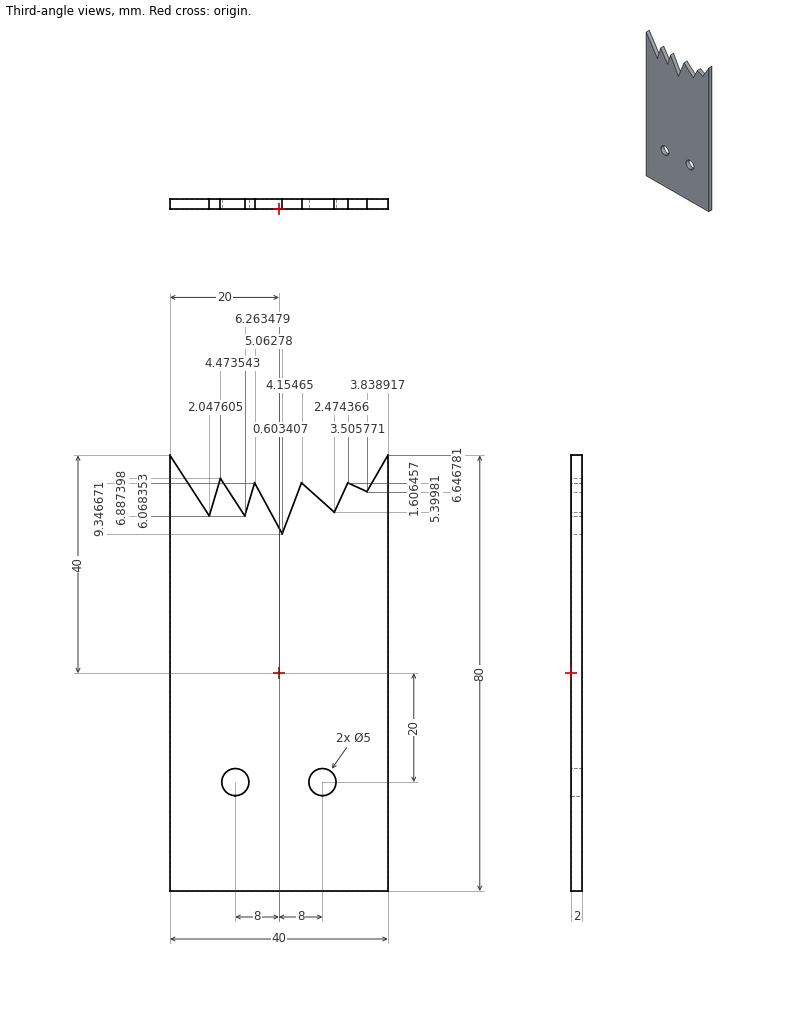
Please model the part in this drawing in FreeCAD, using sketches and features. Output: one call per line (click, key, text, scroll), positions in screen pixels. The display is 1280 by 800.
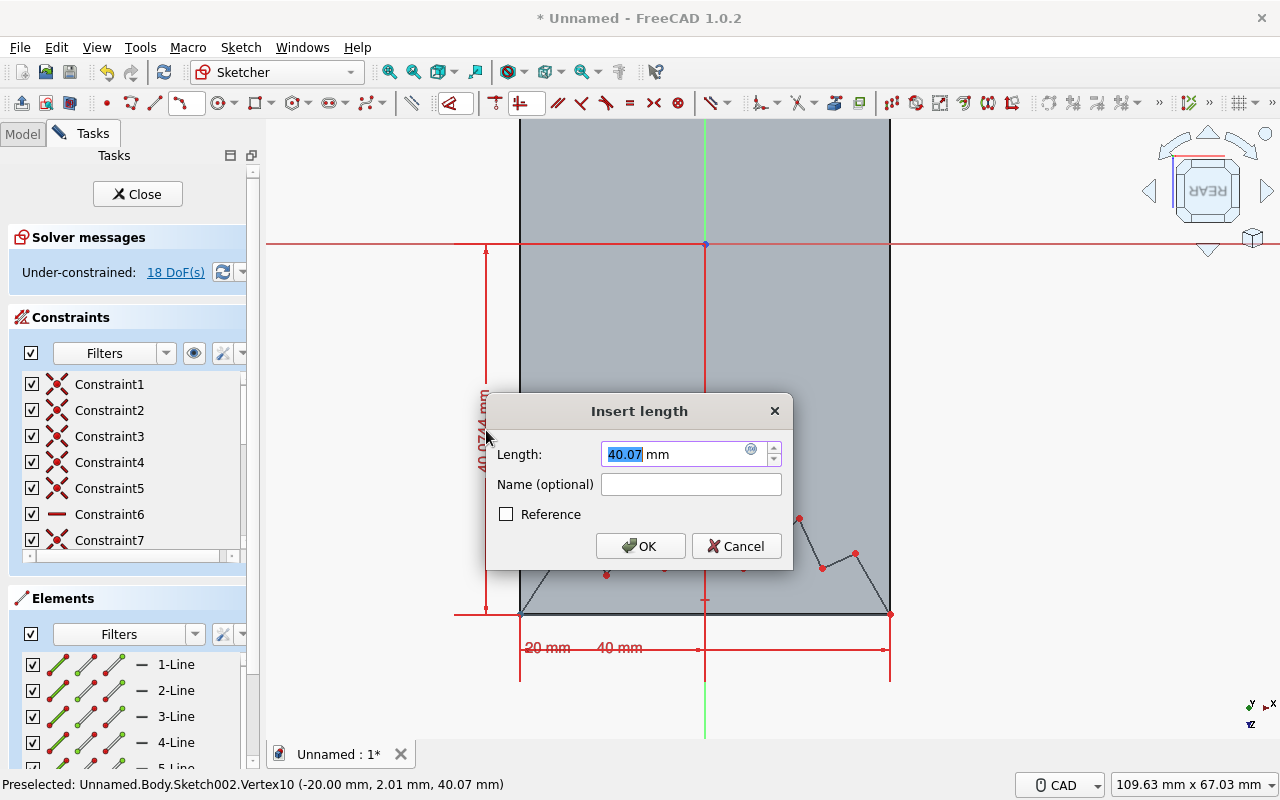
text(40)
key(Return)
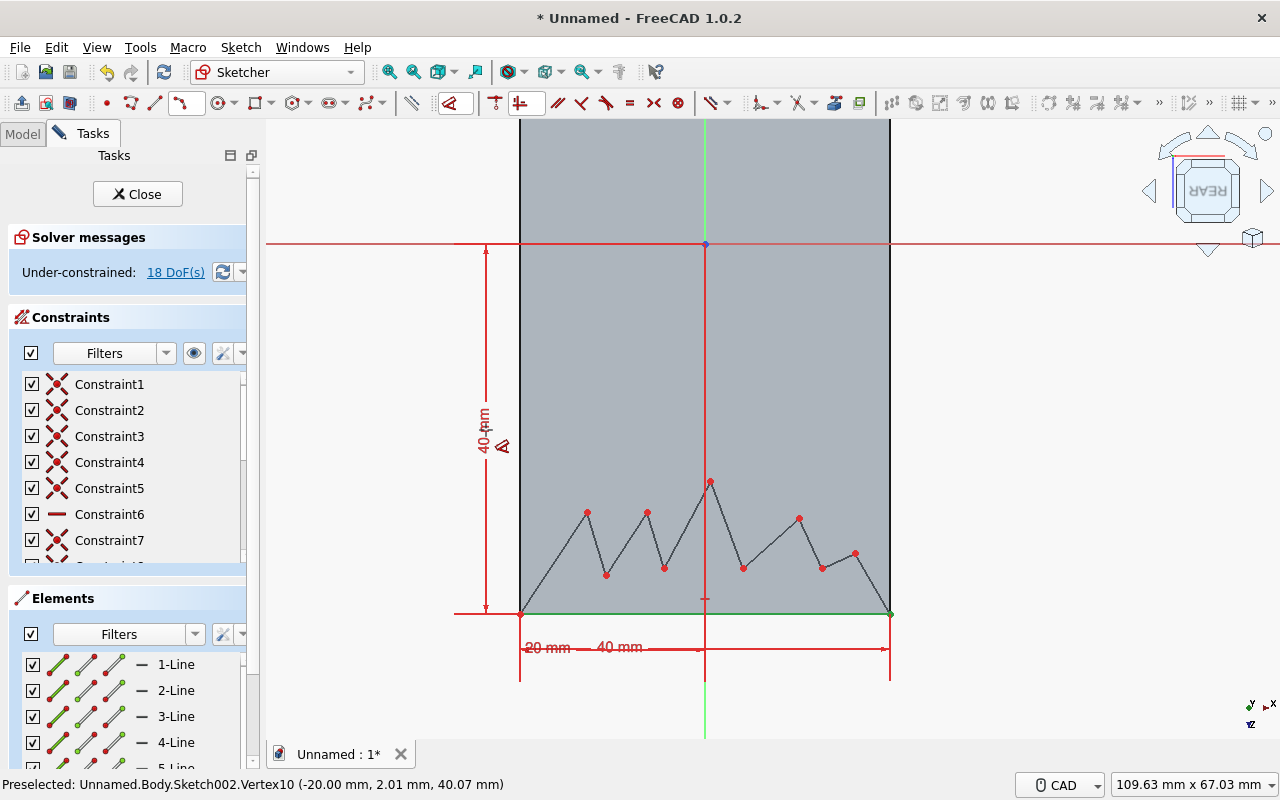
click(743, 569)
click(724, 210)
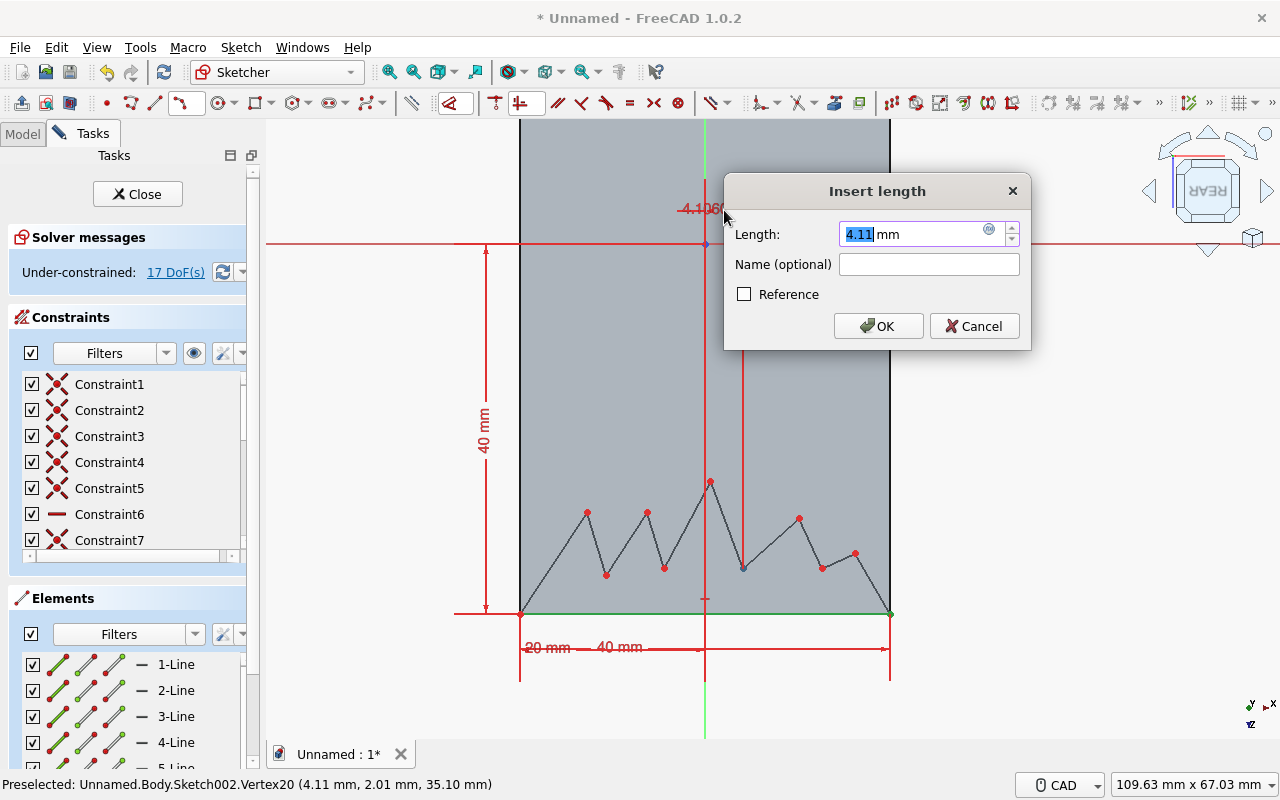
text(4.15465)
key(Return)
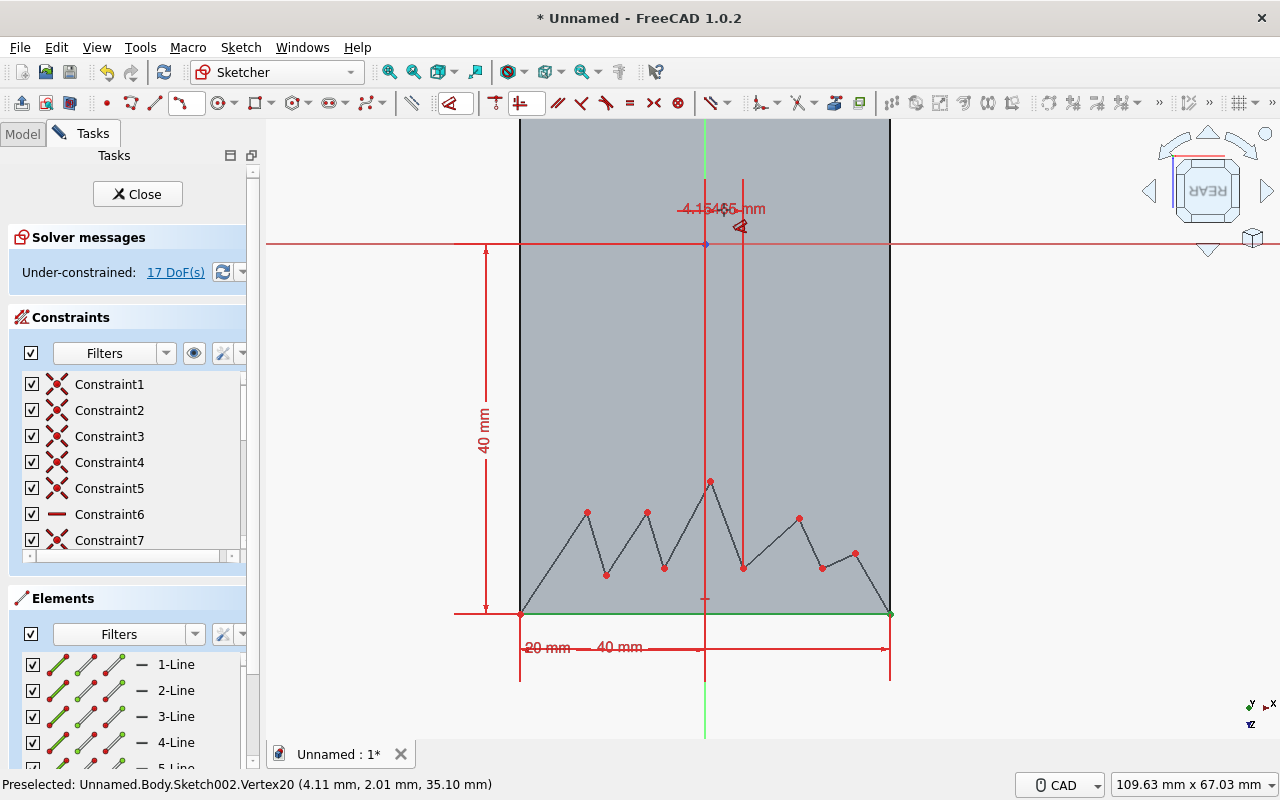
click(678, 543)
click(687, 448)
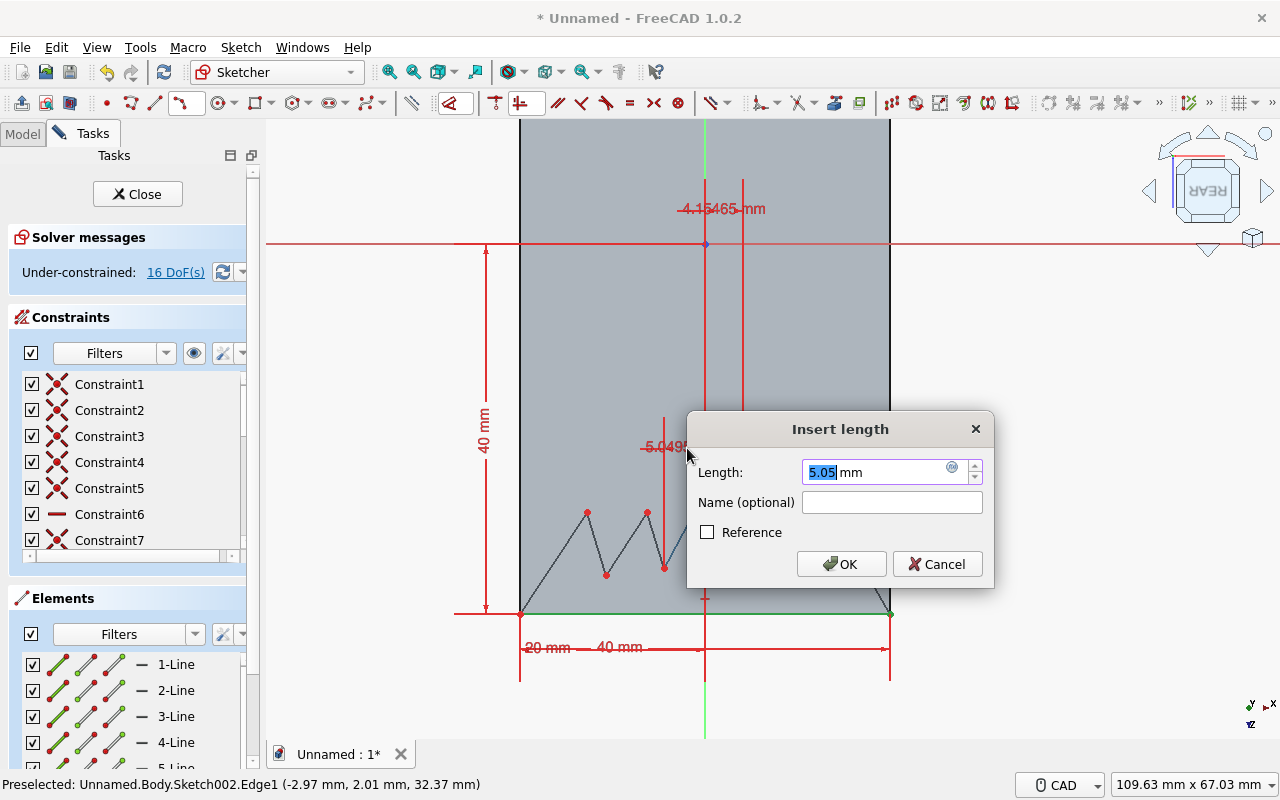
text(5.06278)
key(Return)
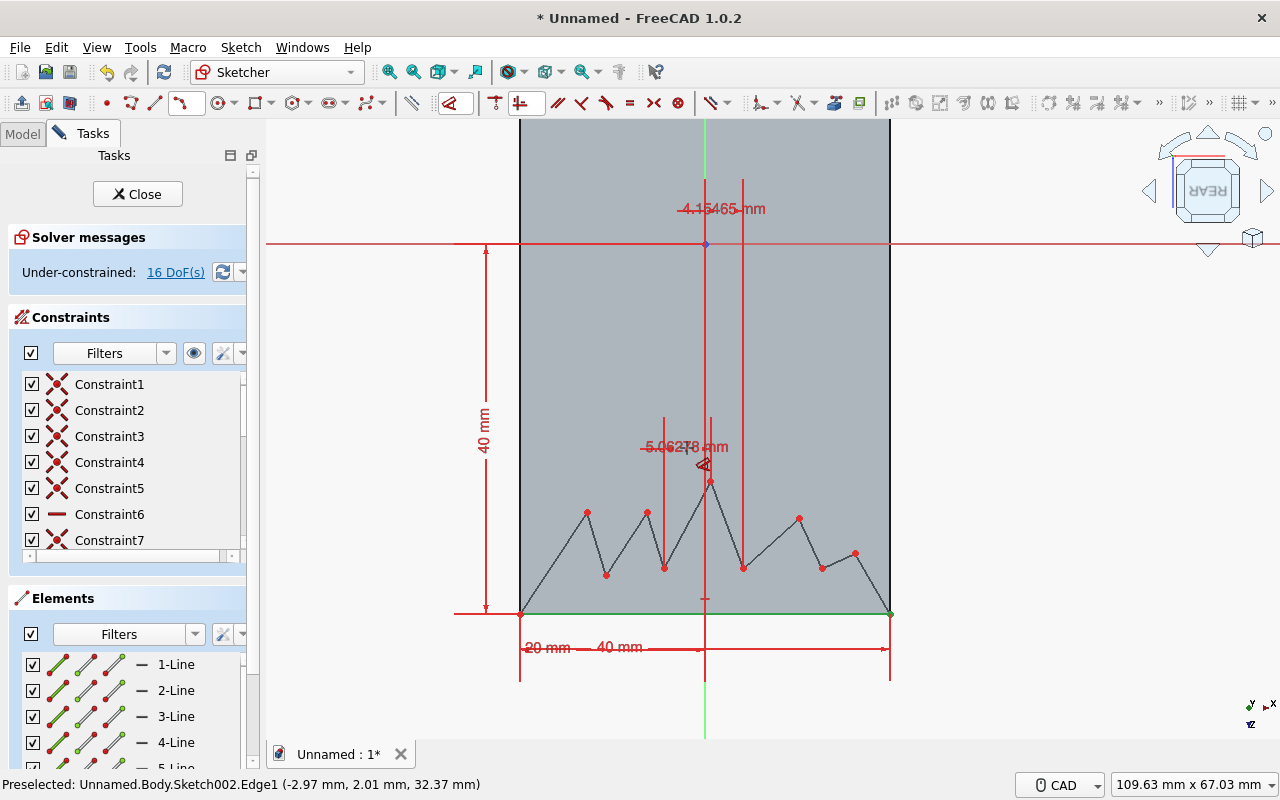
click(815, 554)
click(856, 532)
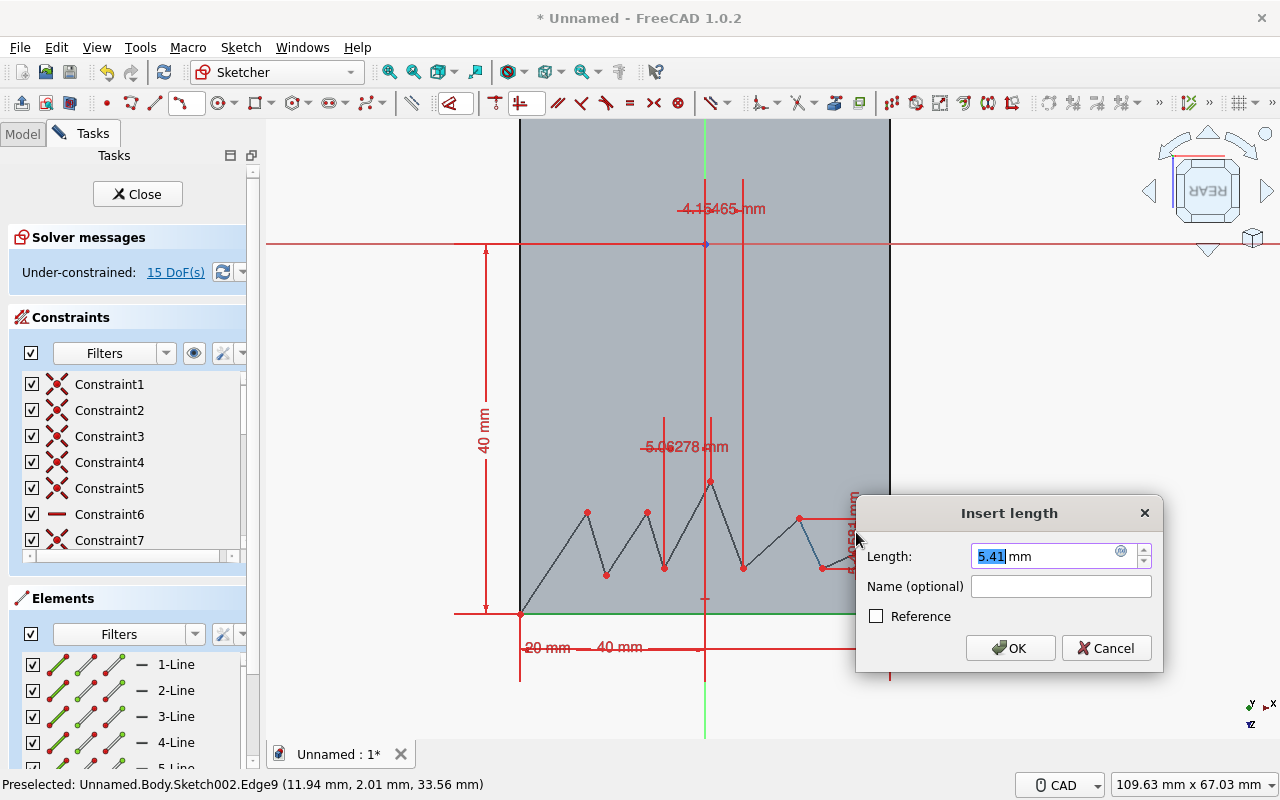
text(5.39981)
key(Return)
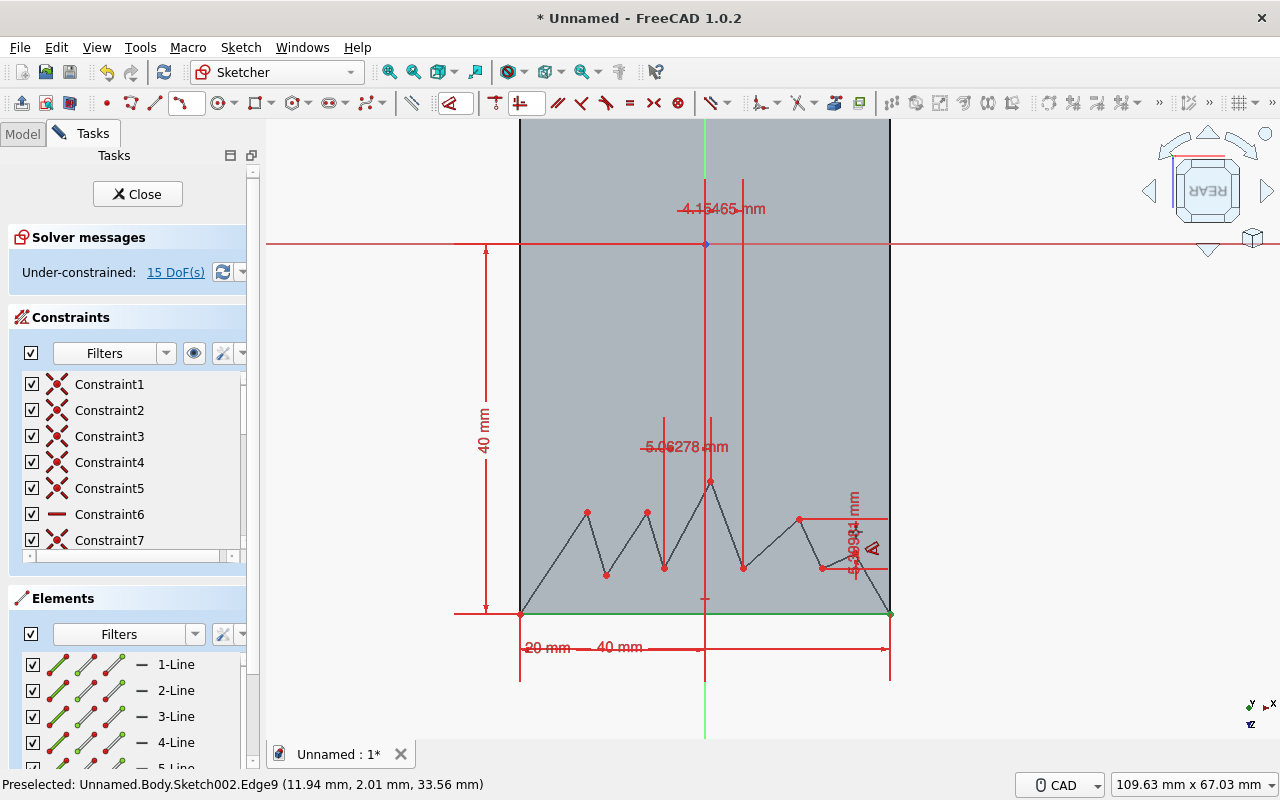
click(782, 534)
click(685, 562)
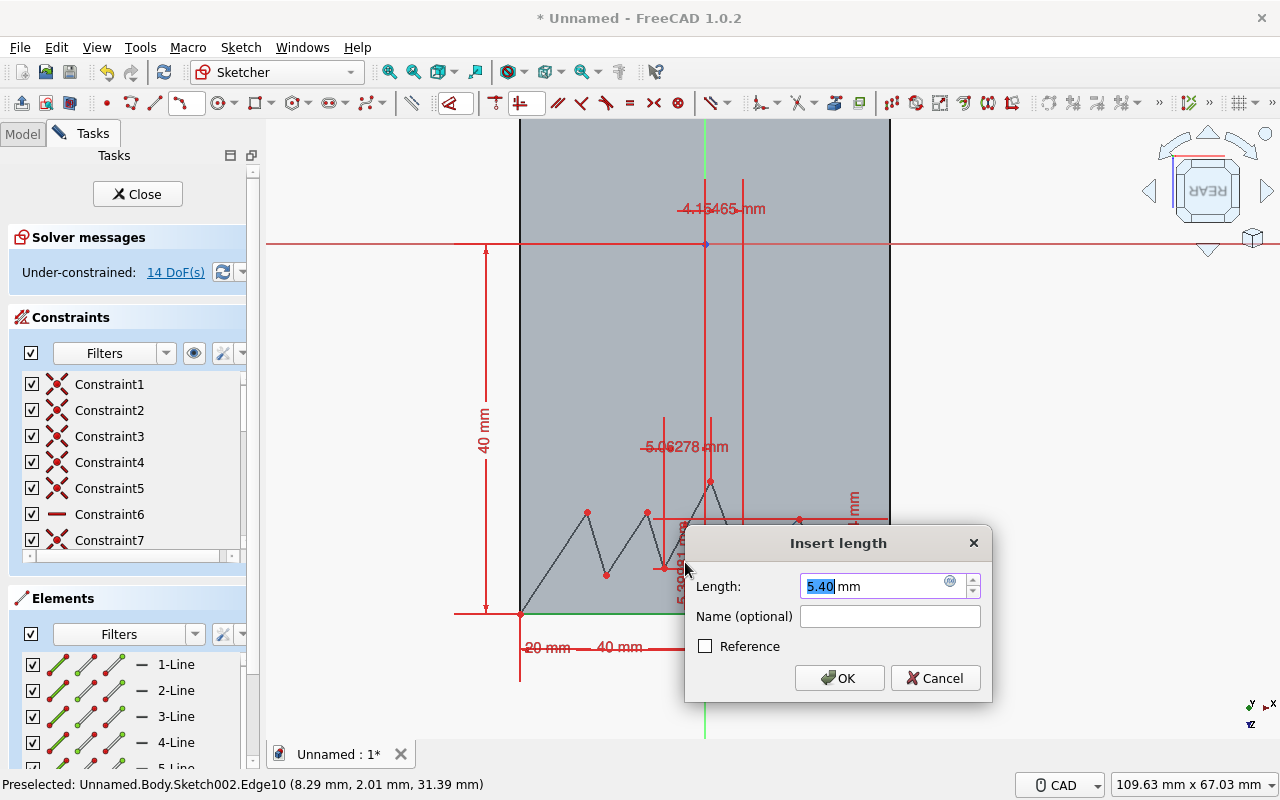
text(5.39981)
key(Return)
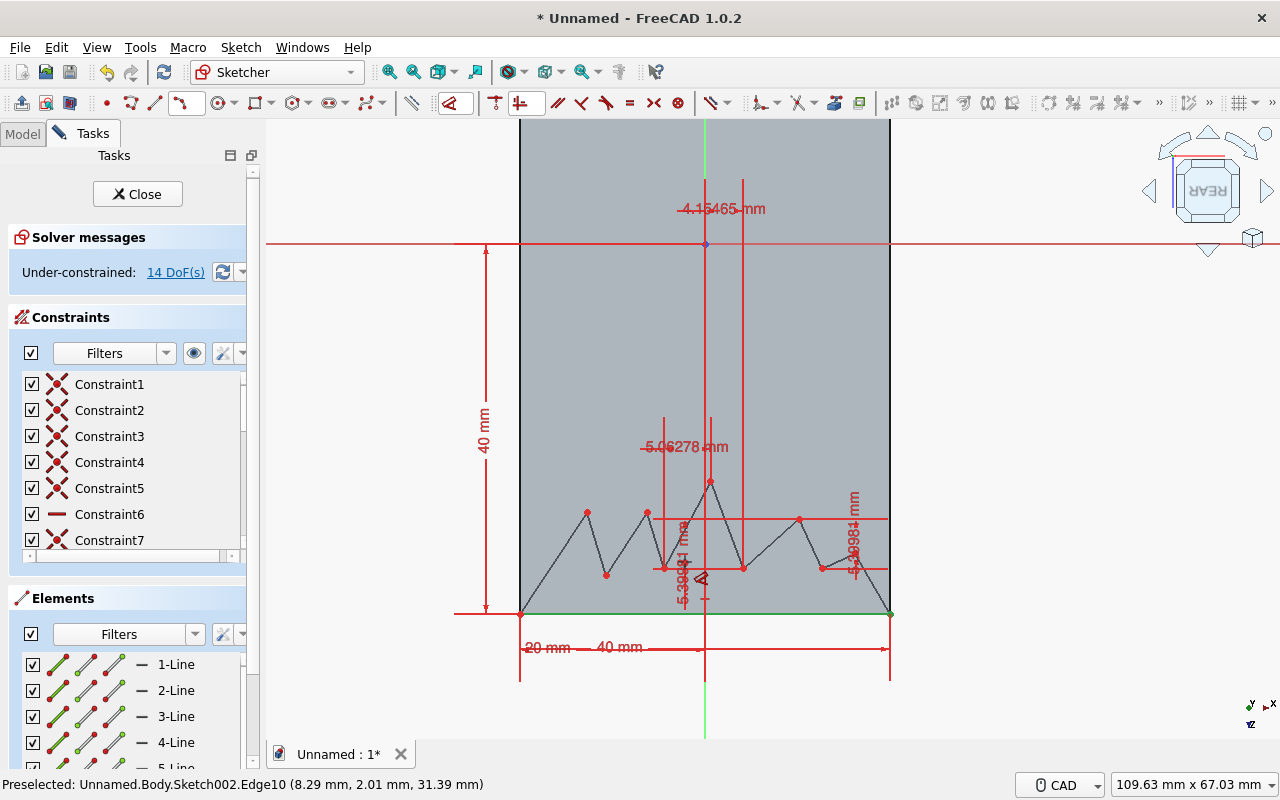
scroll(711, 482, up, 10)